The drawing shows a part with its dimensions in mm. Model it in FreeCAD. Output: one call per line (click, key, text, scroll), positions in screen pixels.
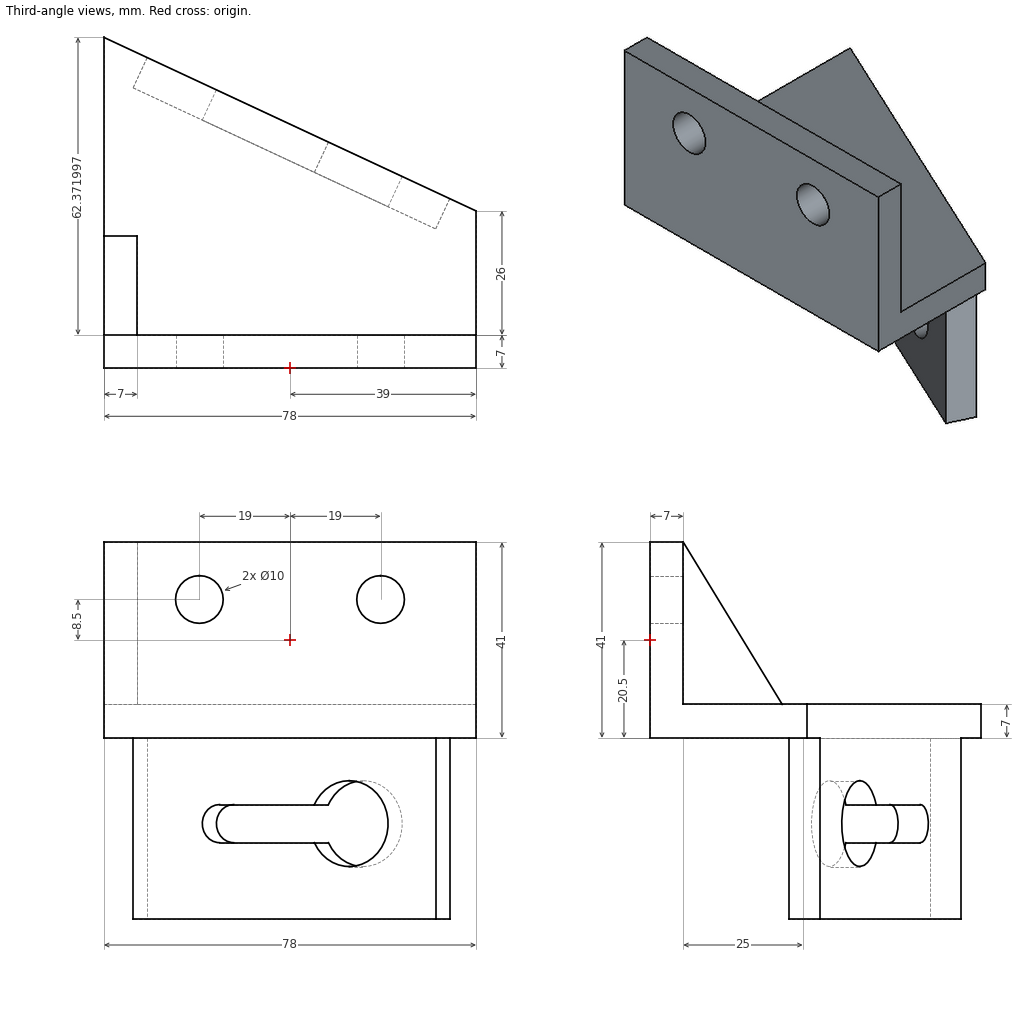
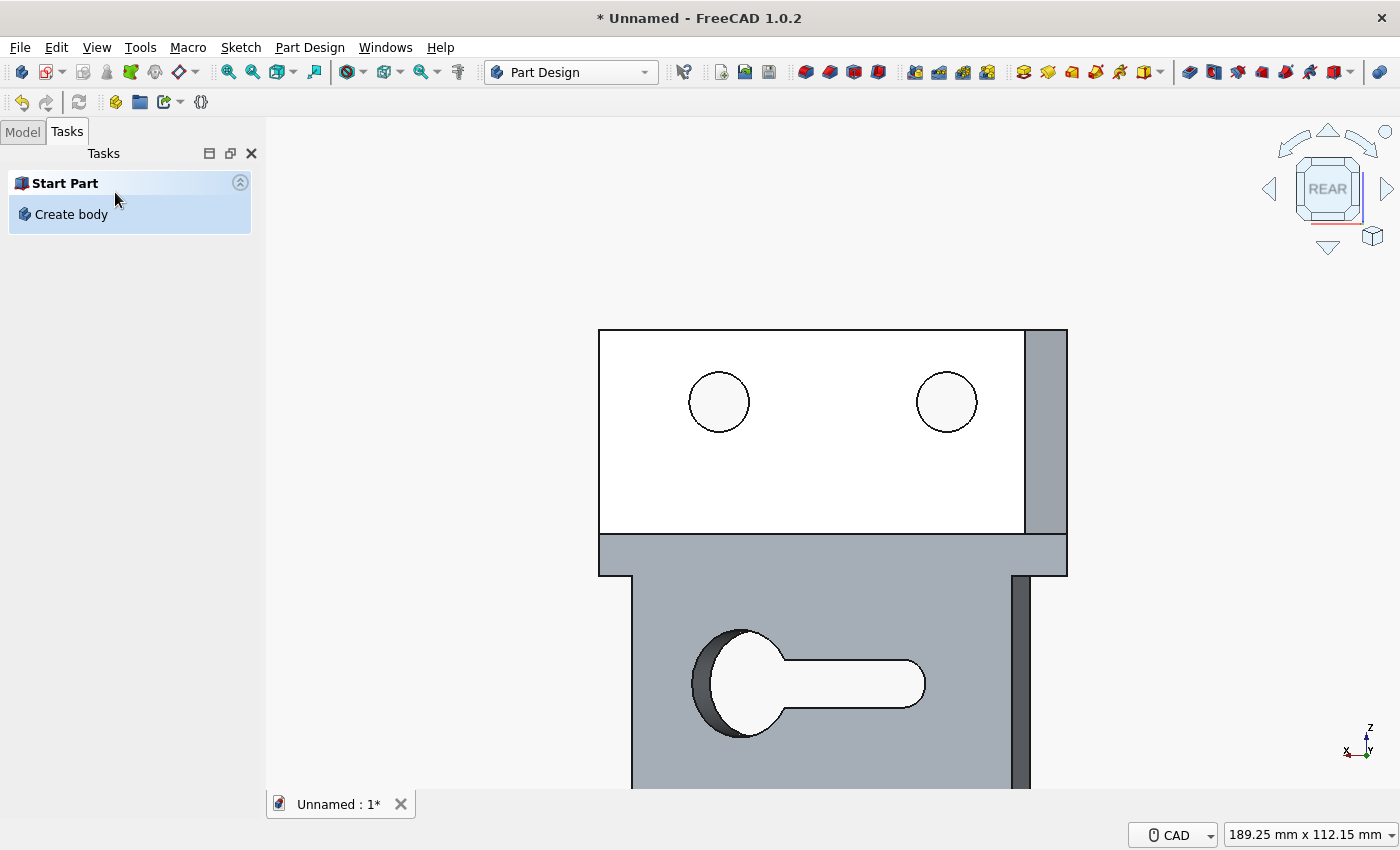
key(0)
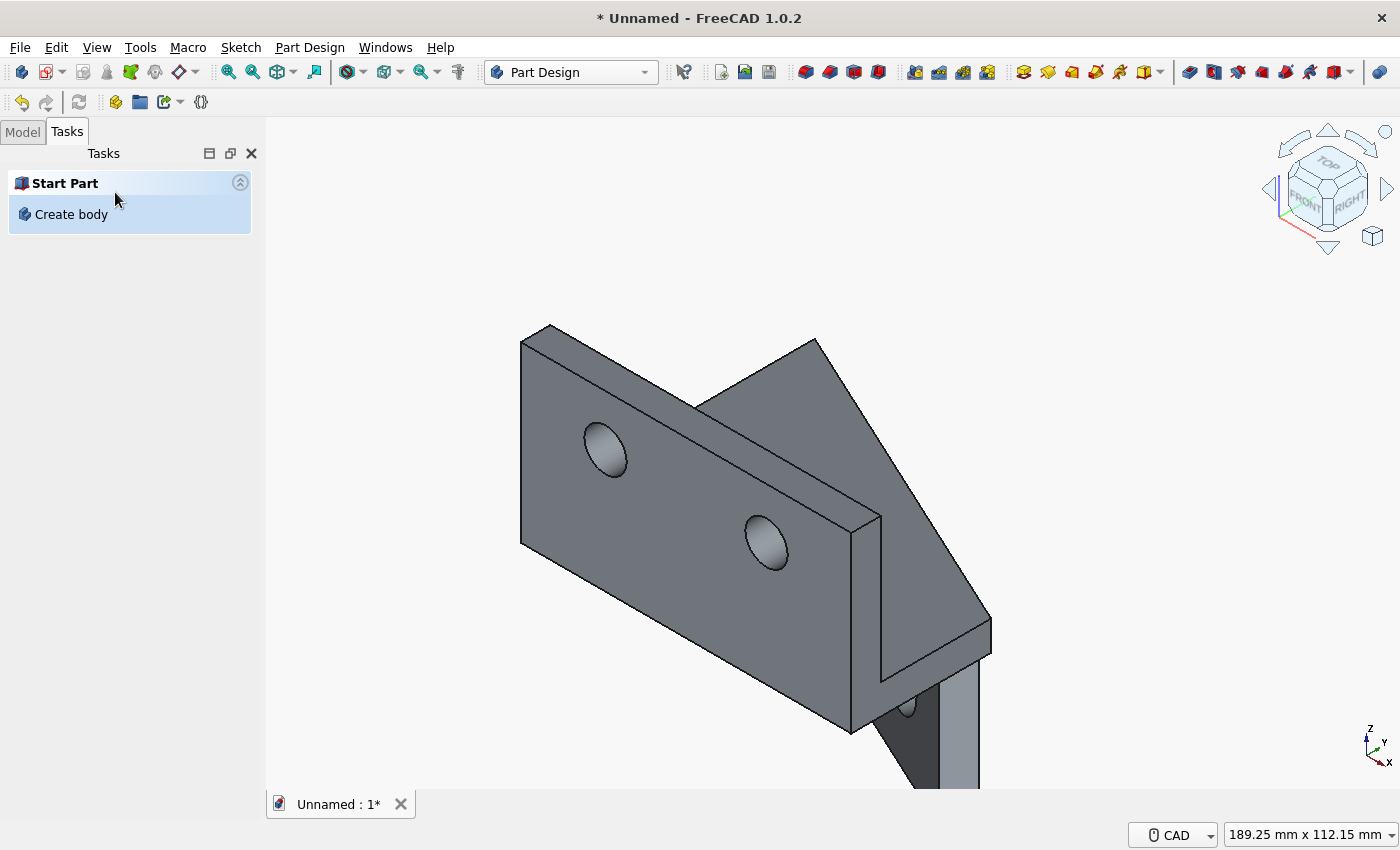
click(230, 72)